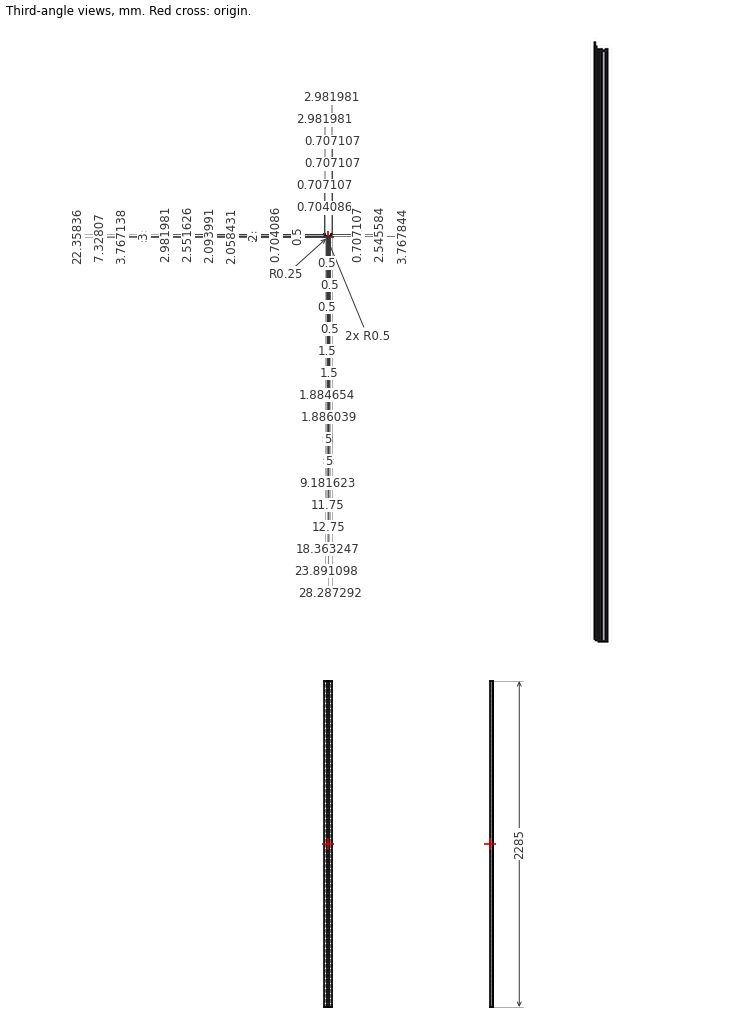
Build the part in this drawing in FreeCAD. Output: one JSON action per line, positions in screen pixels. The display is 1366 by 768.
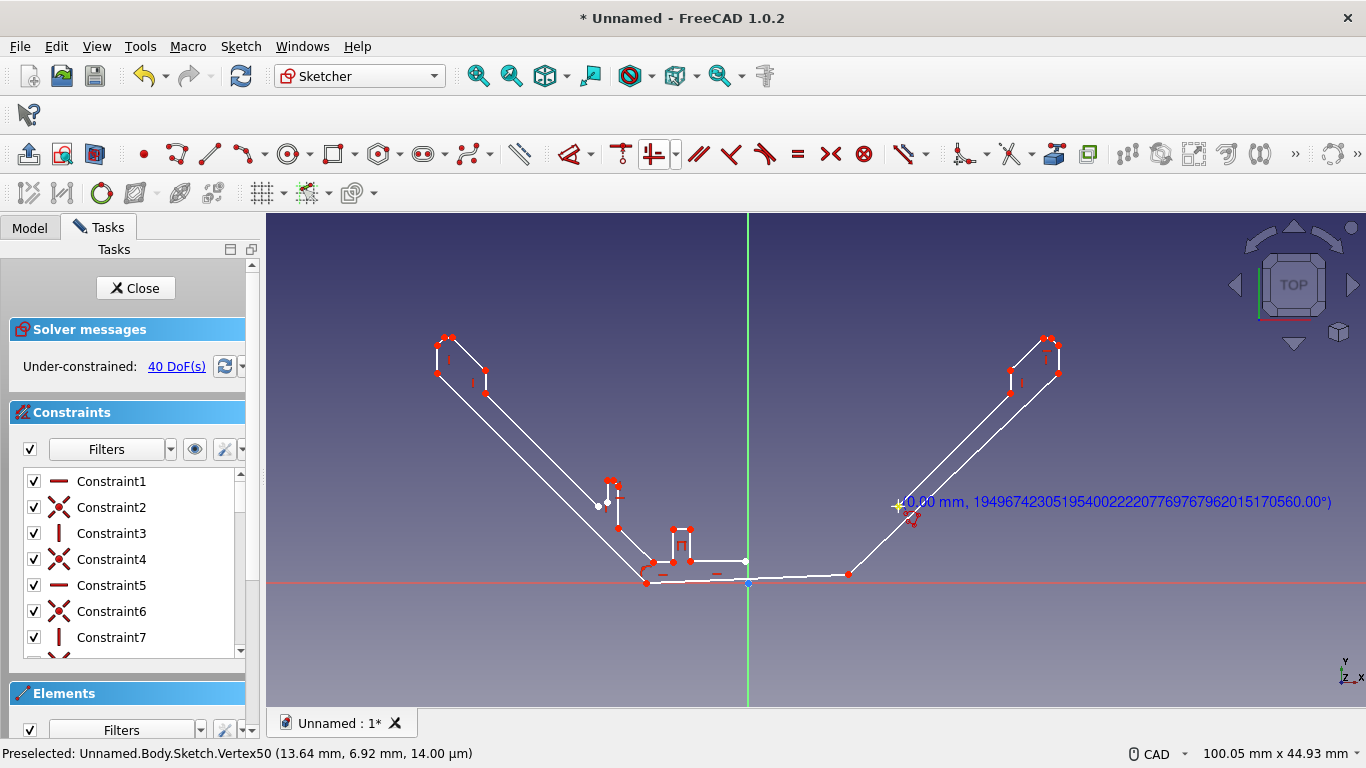
{"action": "scroll", "coordinate": [888, 503], "scroll_direction": "up", "scroll_amount": 3}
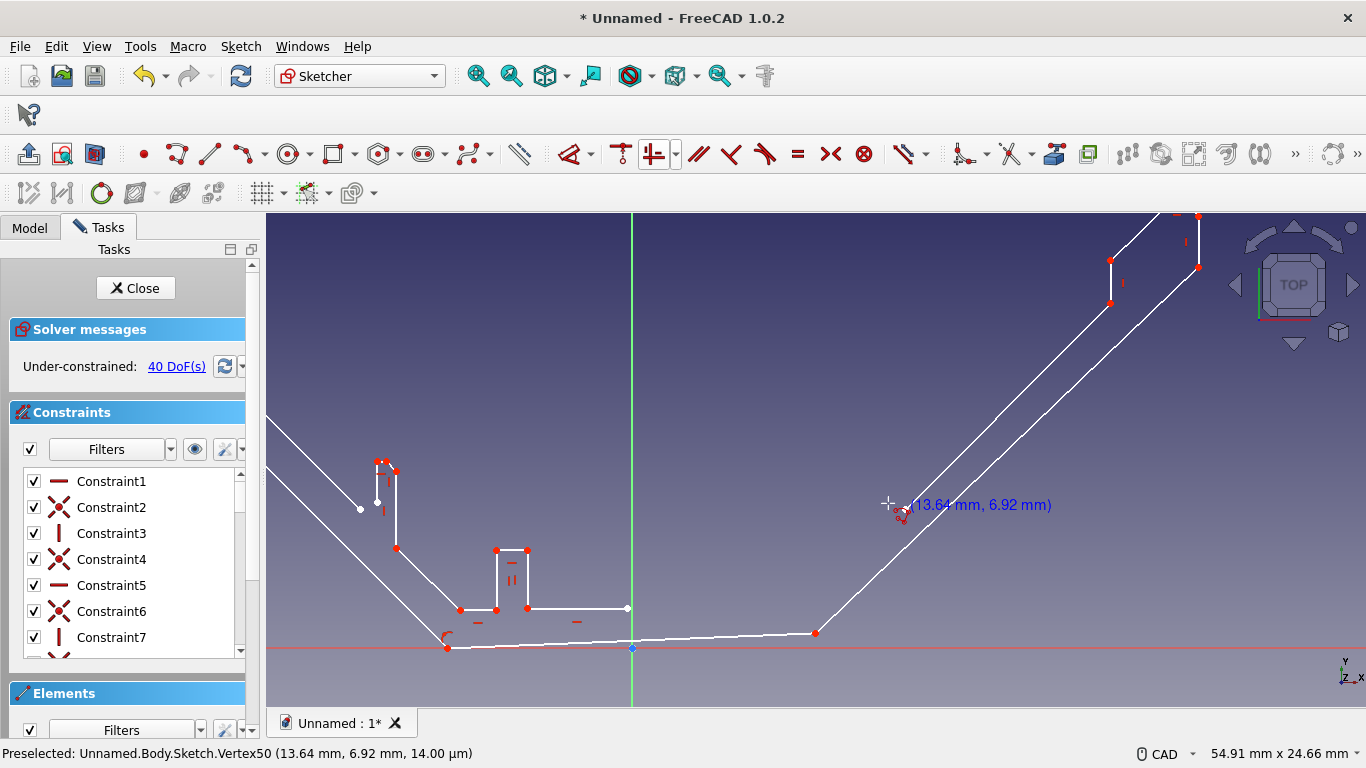
{"action": "left_click", "coordinate": [888, 502]}
{"action": "left_click", "coordinate": [888, 460]}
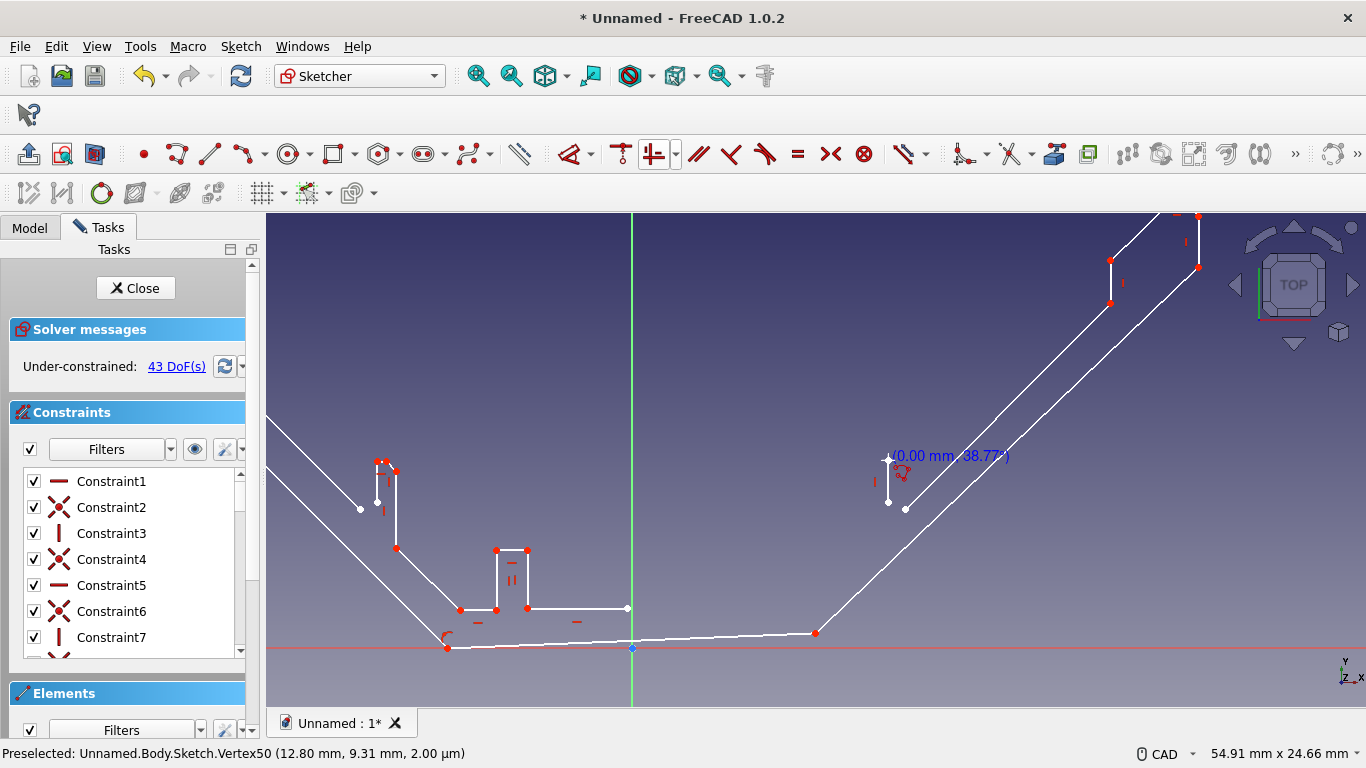
{"action": "scroll", "coordinate": [878, 460], "scroll_direction": "up", "scroll_amount": 3}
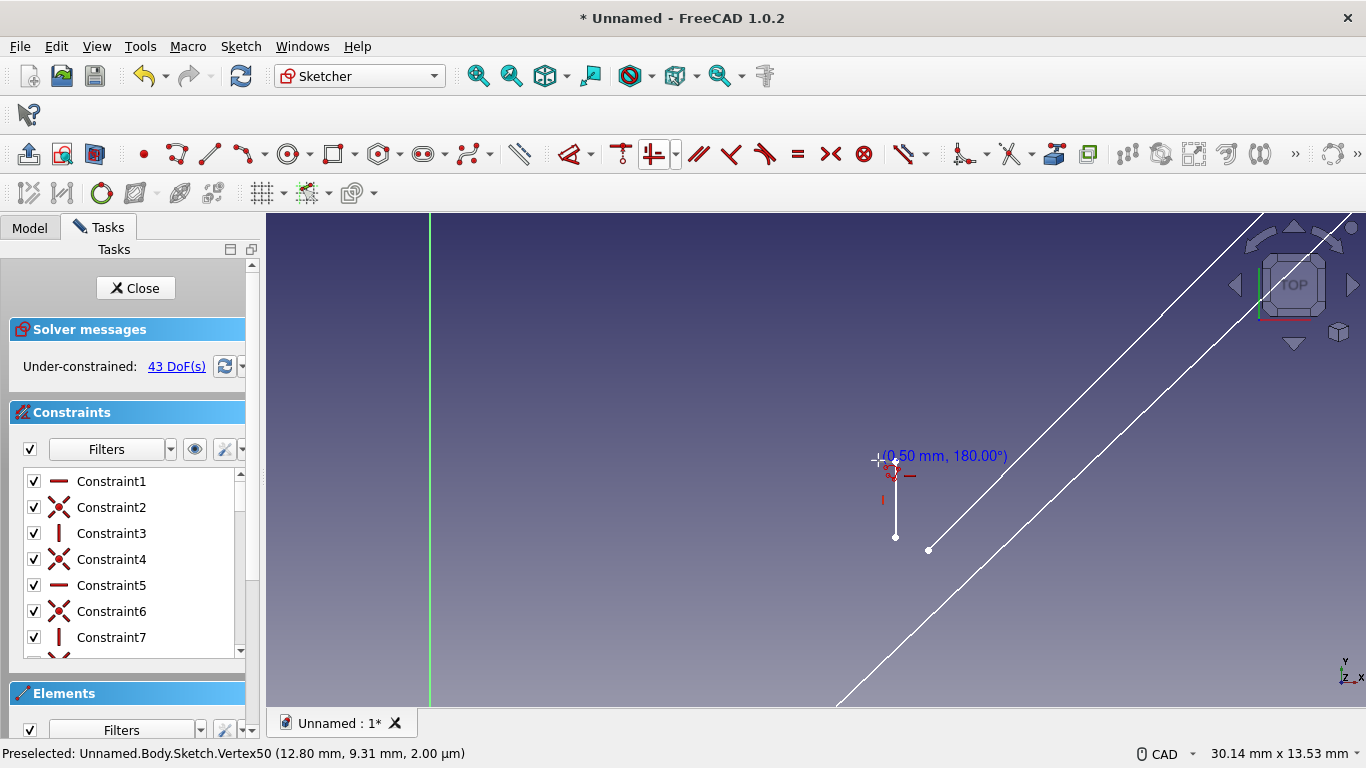
{"action": "left_click", "coordinate": [877, 460]}
{"action": "left_click", "coordinate": [859, 479]}
{"action": "left_click", "coordinate": [859, 616]}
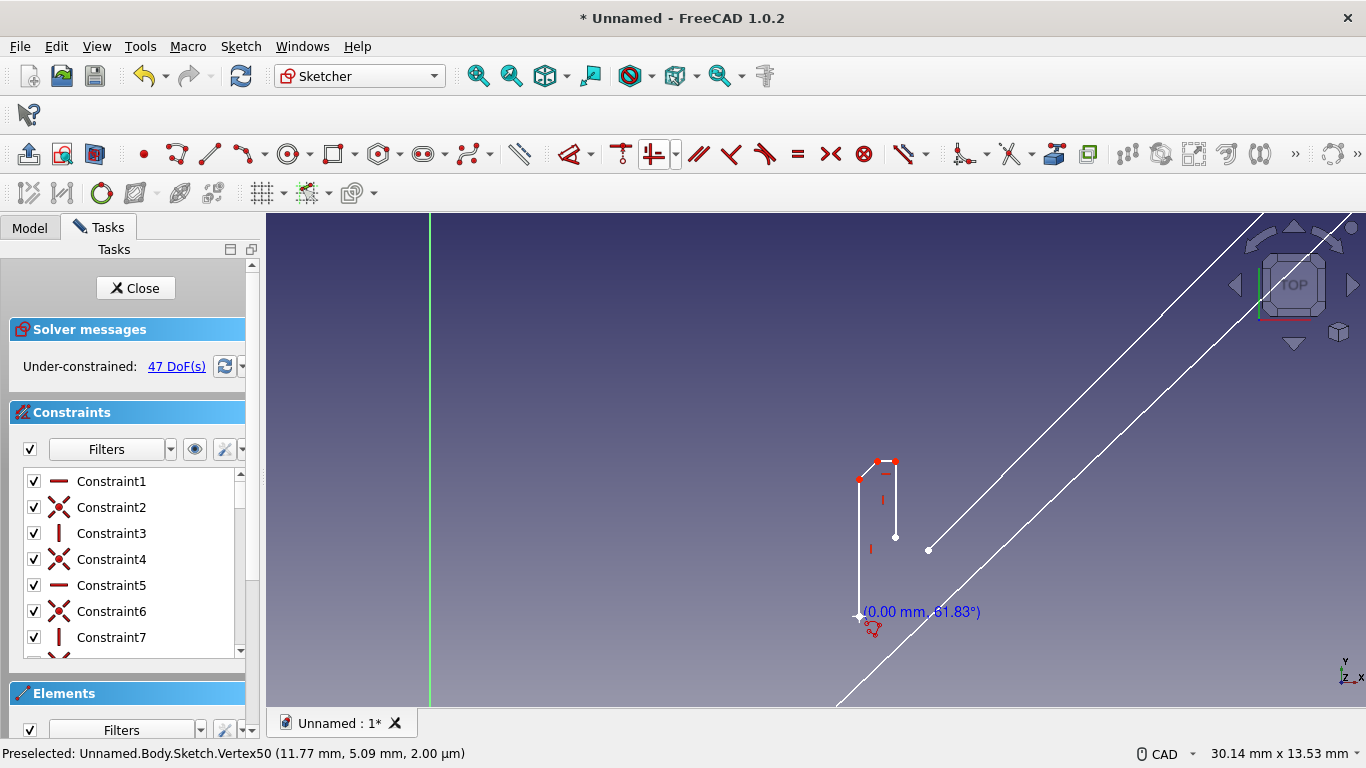
{"action": "scroll", "coordinate": [884, 488], "scroll_direction": "down", "scroll_amount": 6}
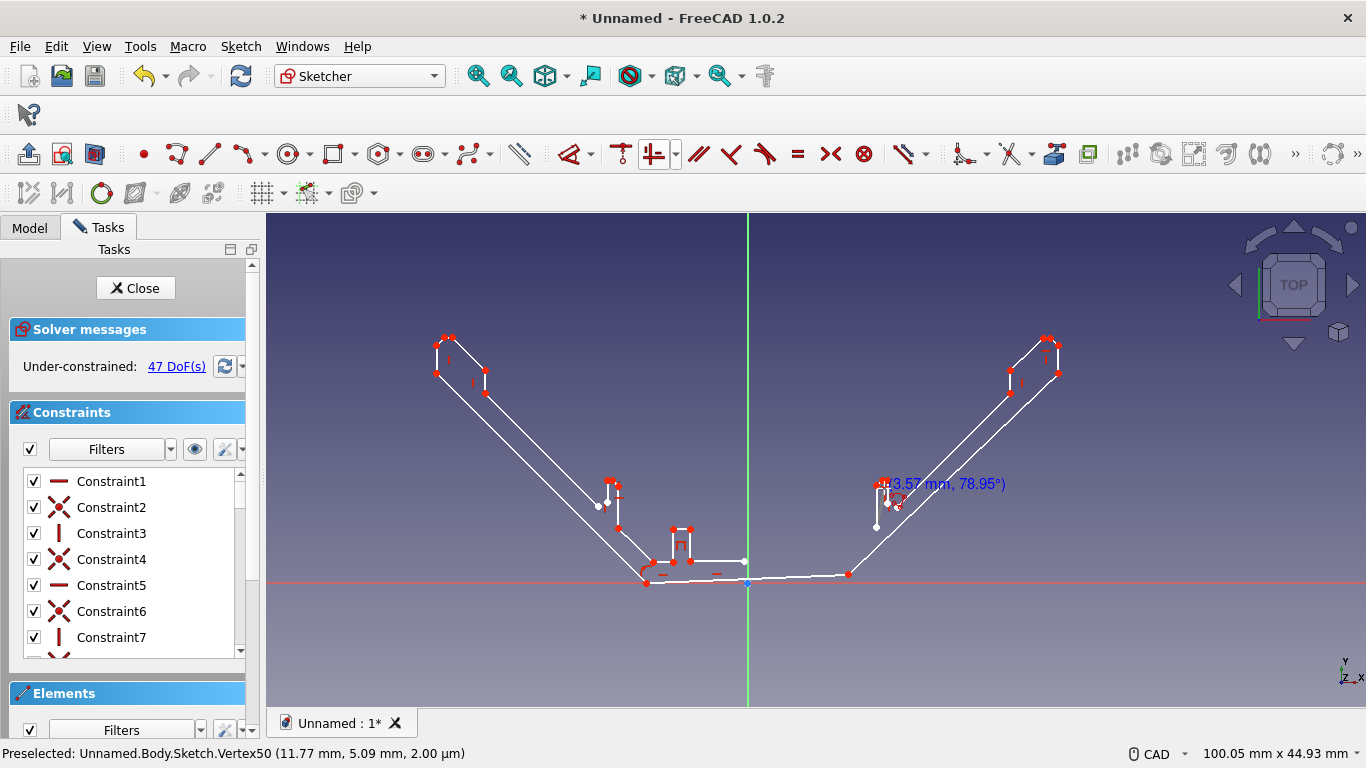
{"action": "left_click", "coordinate": [843, 561]}
{"action": "left_click", "coordinate": [822, 561]}
{"action": "left_click", "coordinate": [822, 528]}
{"action": "left_click", "coordinate": [805, 528]}
{"action": "left_click", "coordinate": [805, 561]}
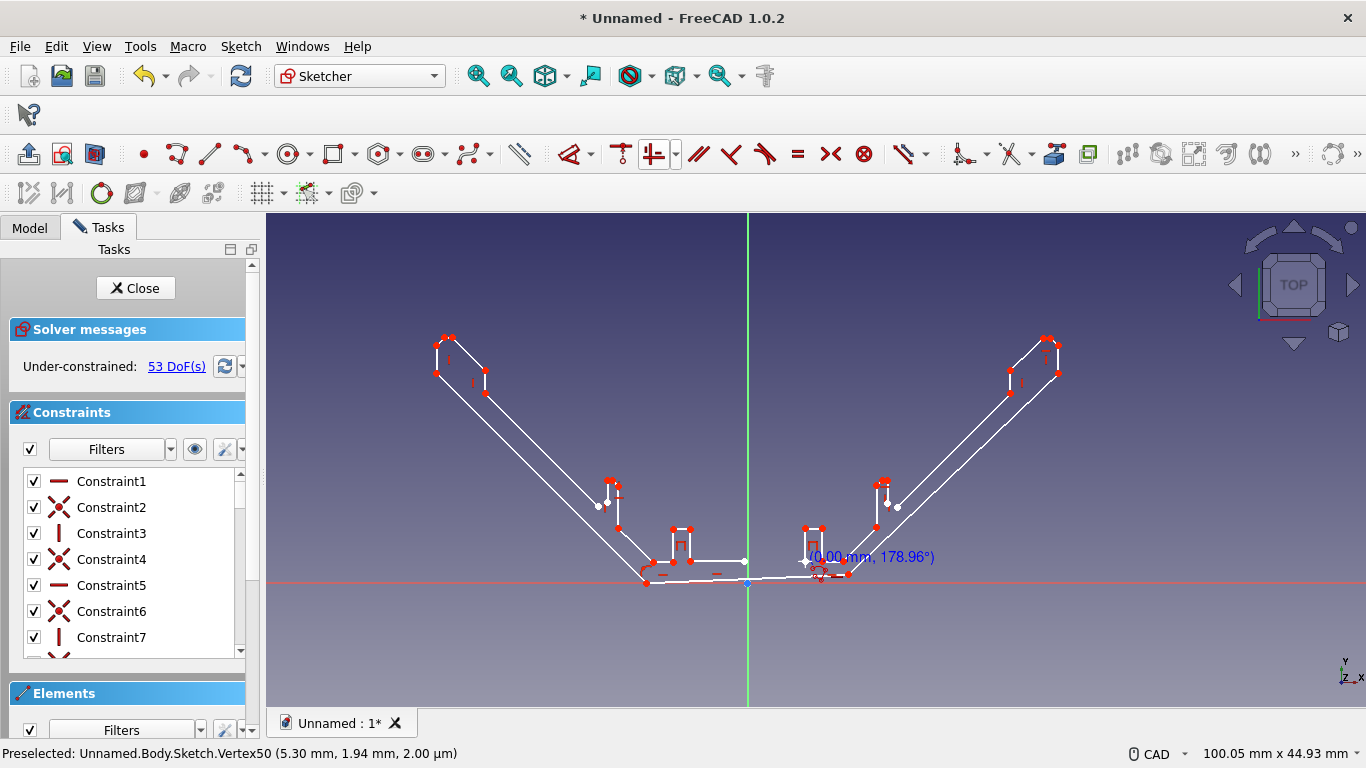
{"action": "scroll", "coordinate": [750, 561], "scroll_direction": "up", "scroll_amount": 9}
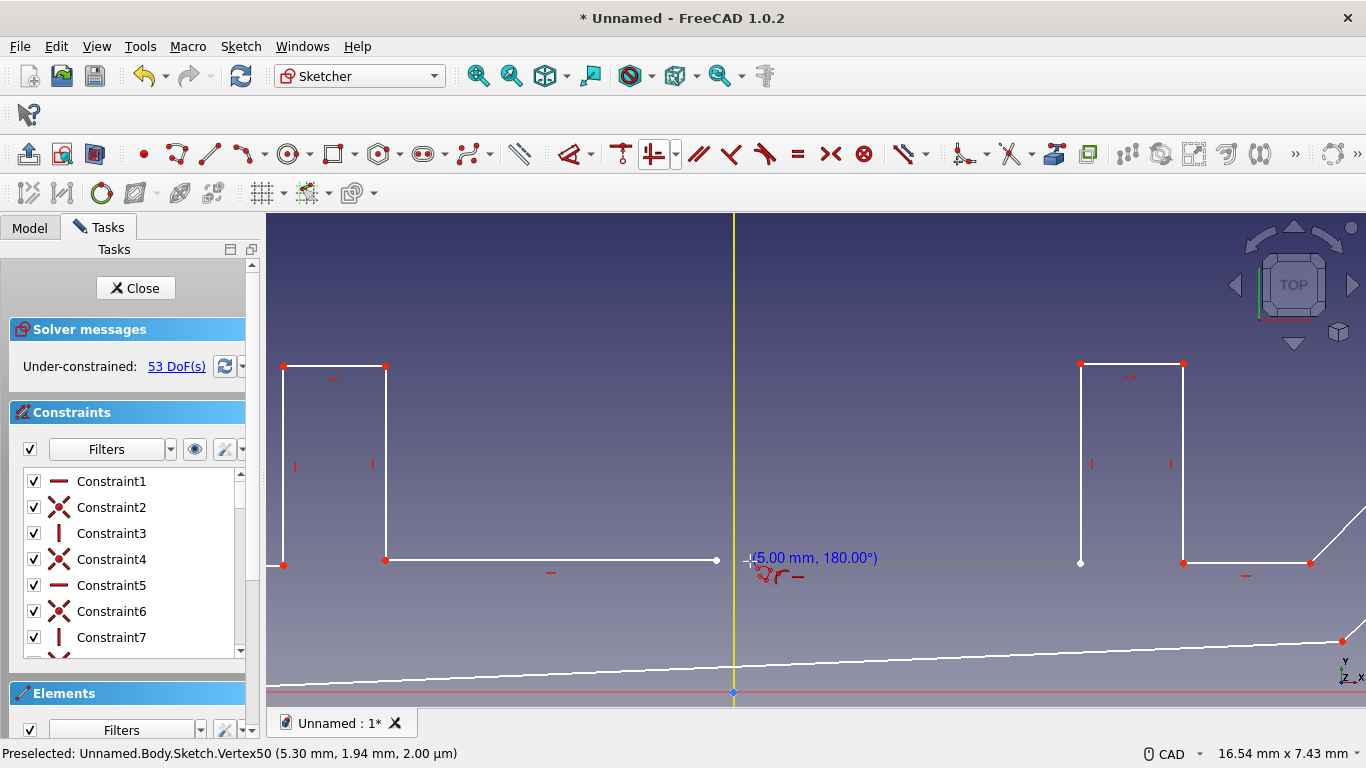
{"action": "left_click", "coordinate": [751, 557]}
{"action": "right_click", "coordinate": [751, 557]}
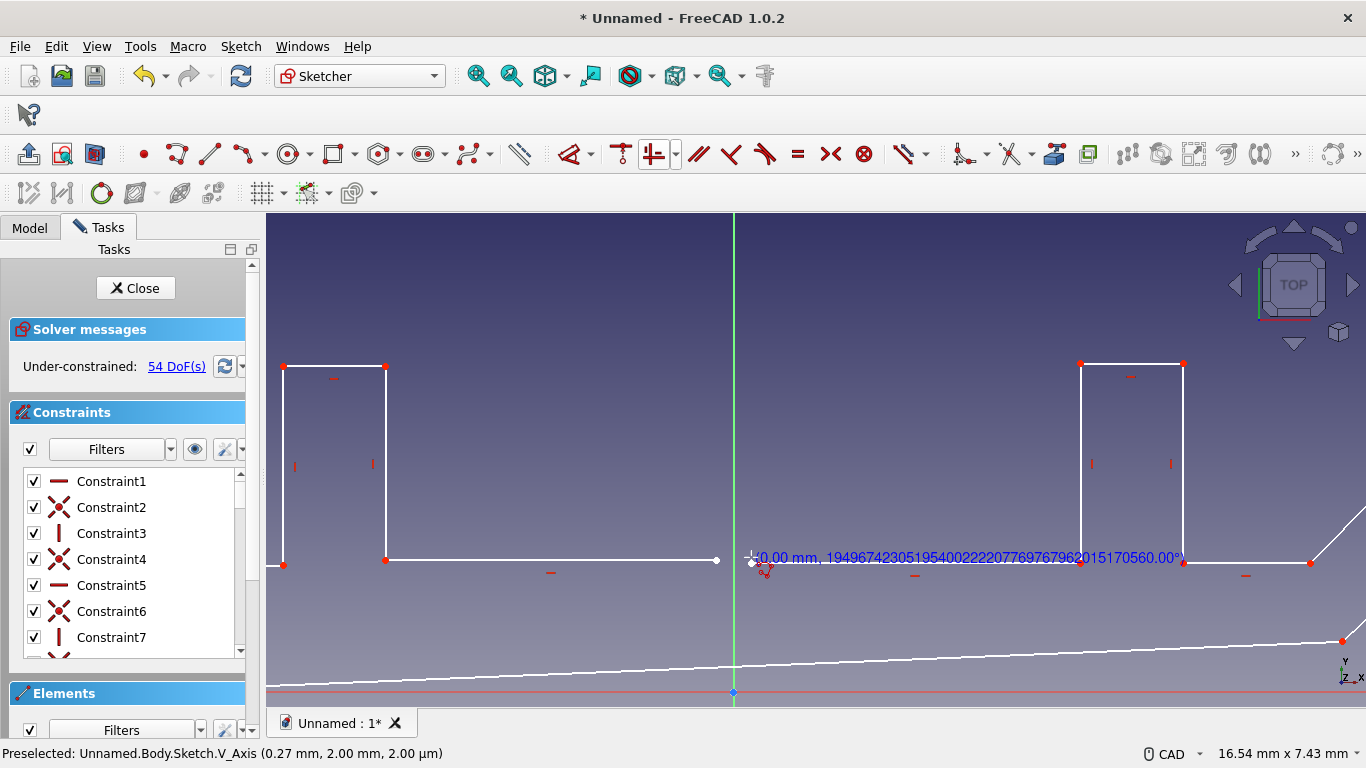
{"action": "left_click", "coordinate": [242, 154]}